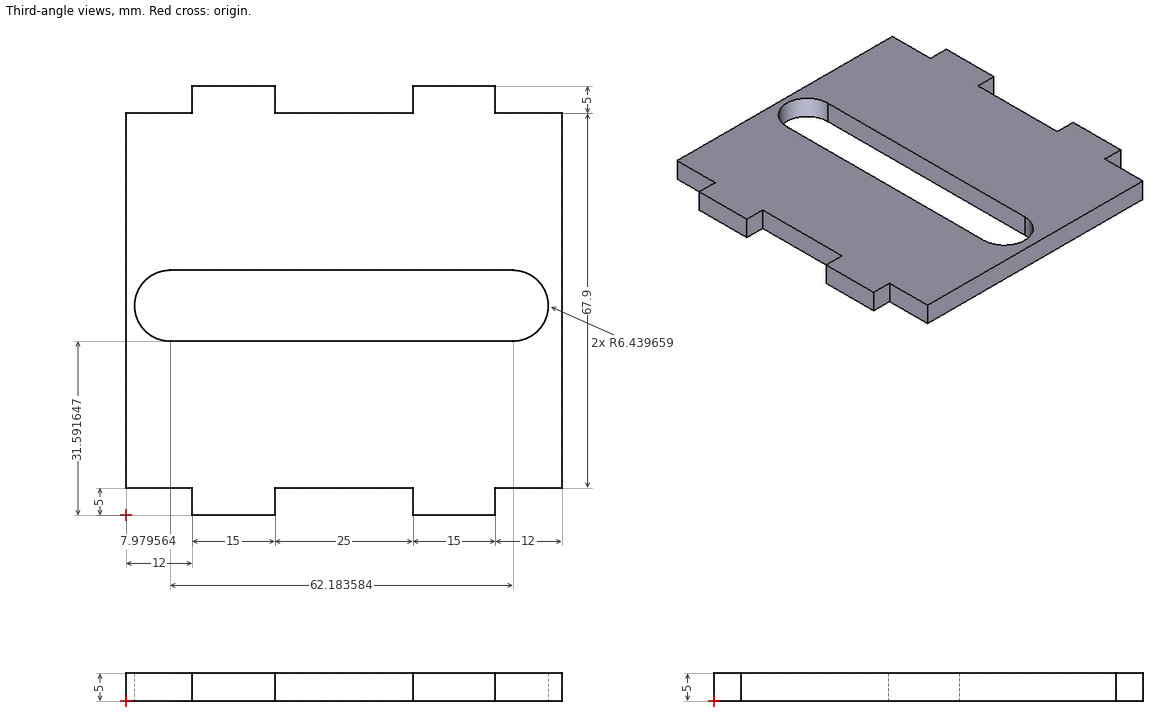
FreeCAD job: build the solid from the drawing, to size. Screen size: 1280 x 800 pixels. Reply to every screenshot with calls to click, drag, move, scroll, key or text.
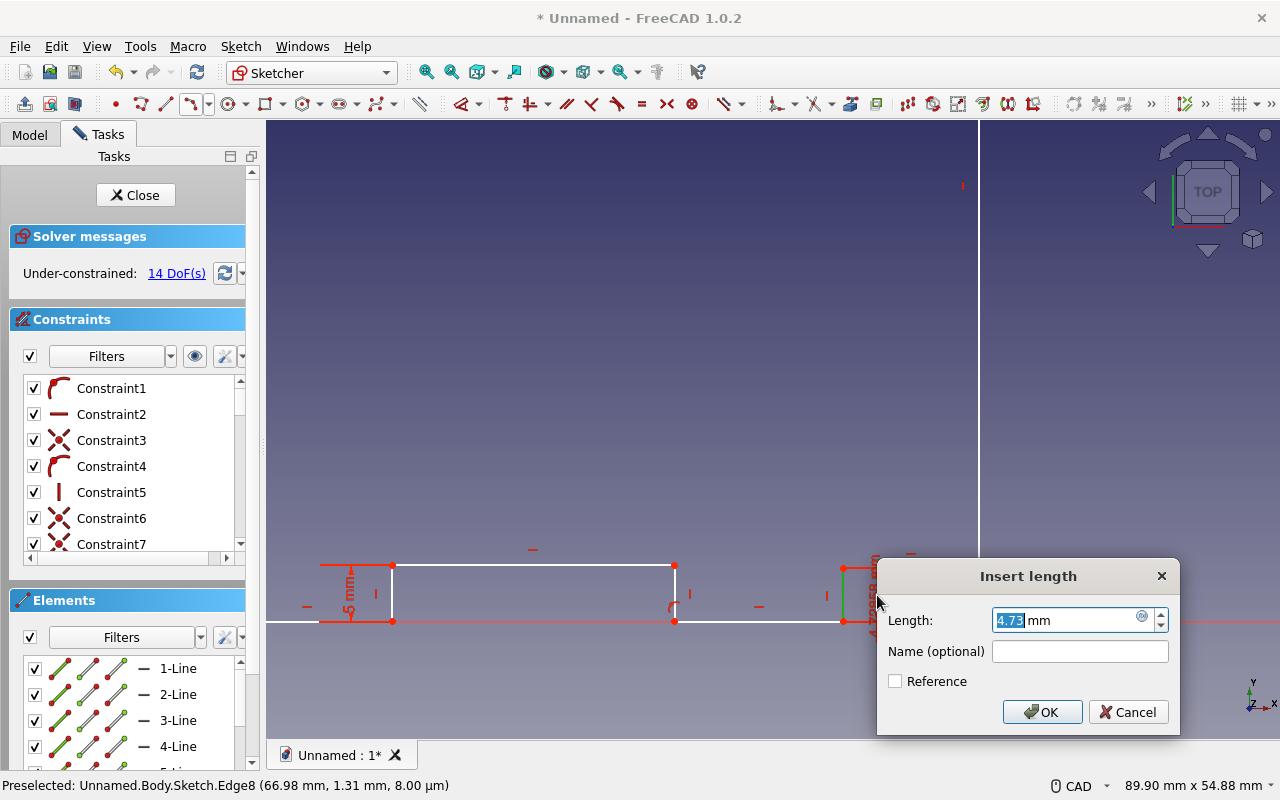
text(5)
key(Return)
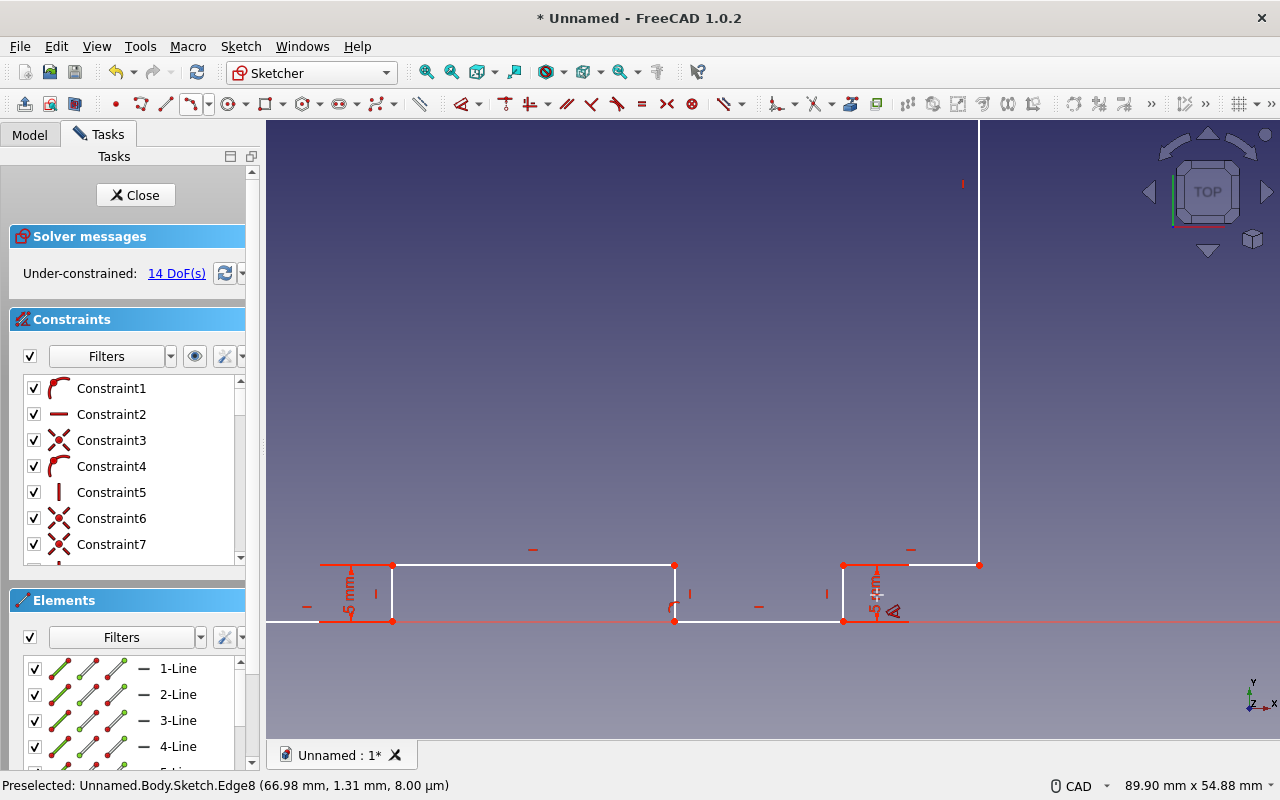
scroll(844, 631, down, 4)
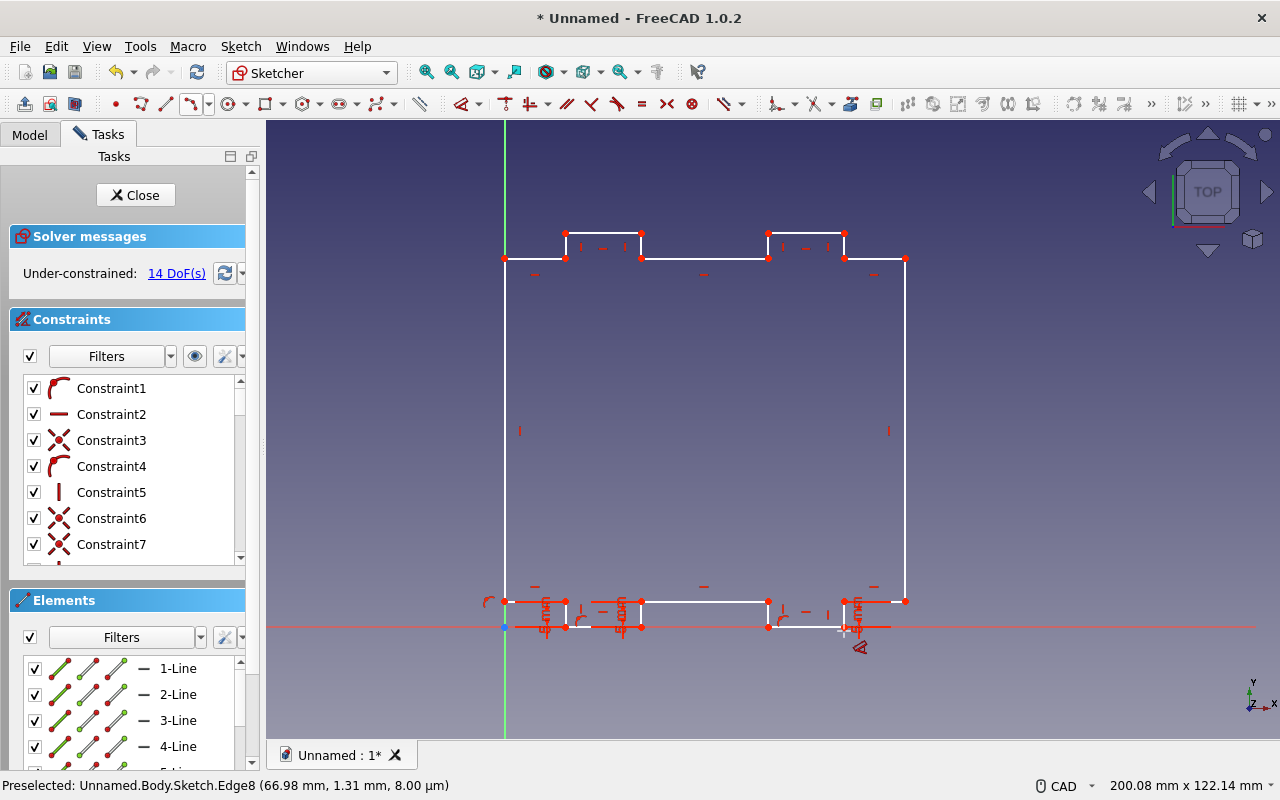
scroll(844, 251, up, 3)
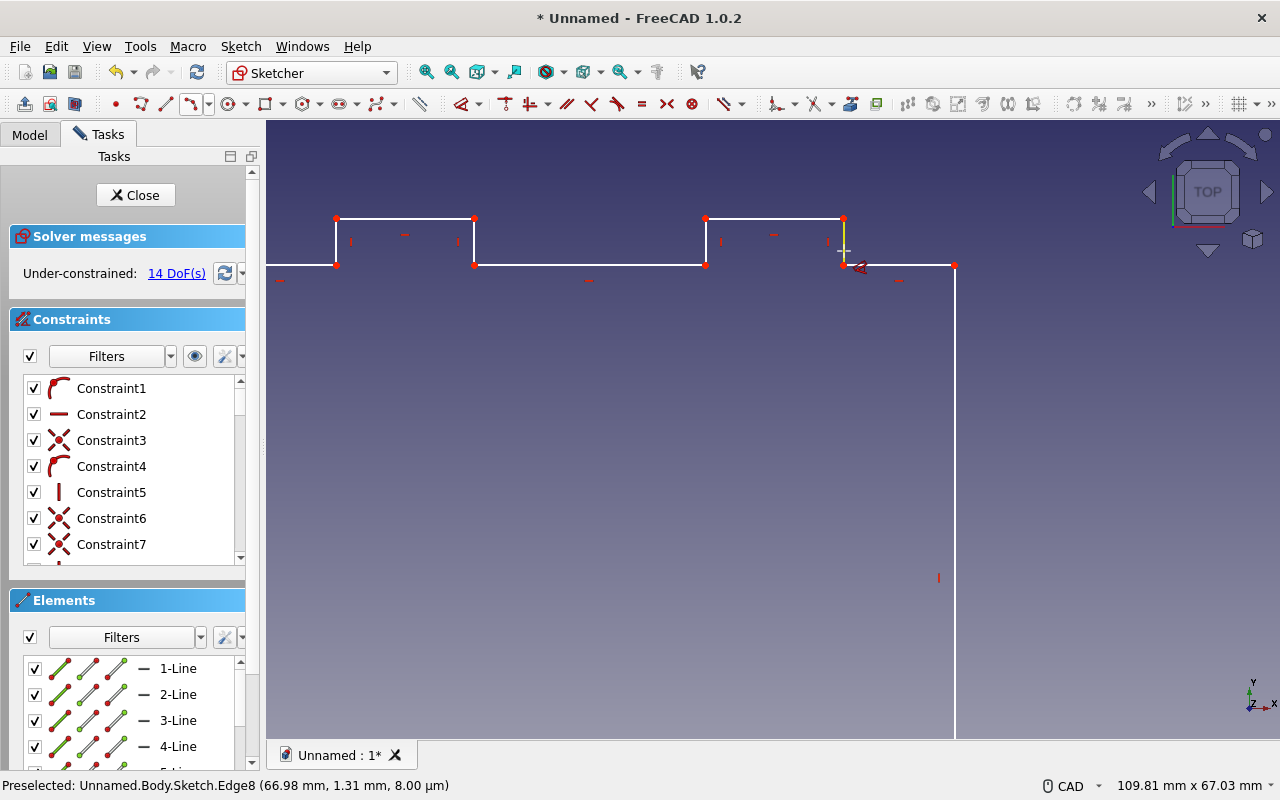
click(844, 251)
click(878, 242)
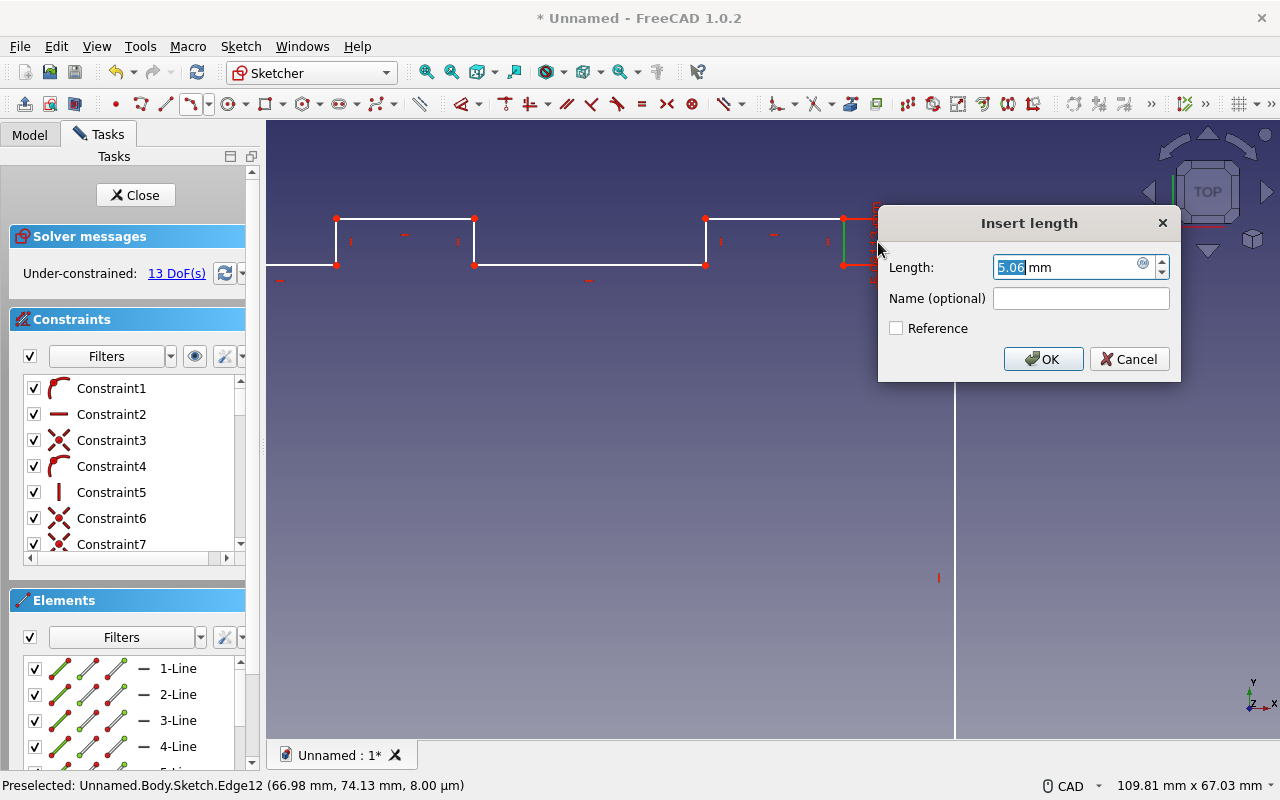
text(5)
key(Return)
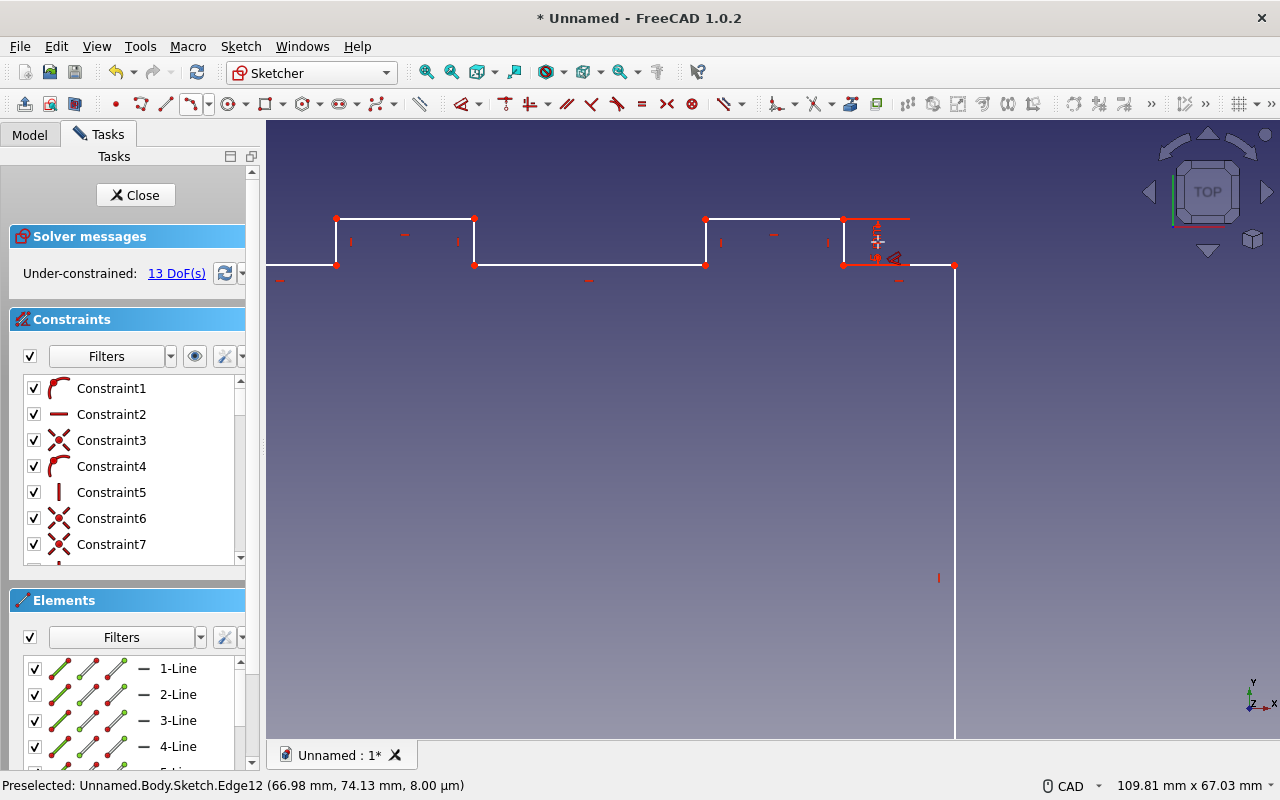
click(706, 233)
click(740, 242)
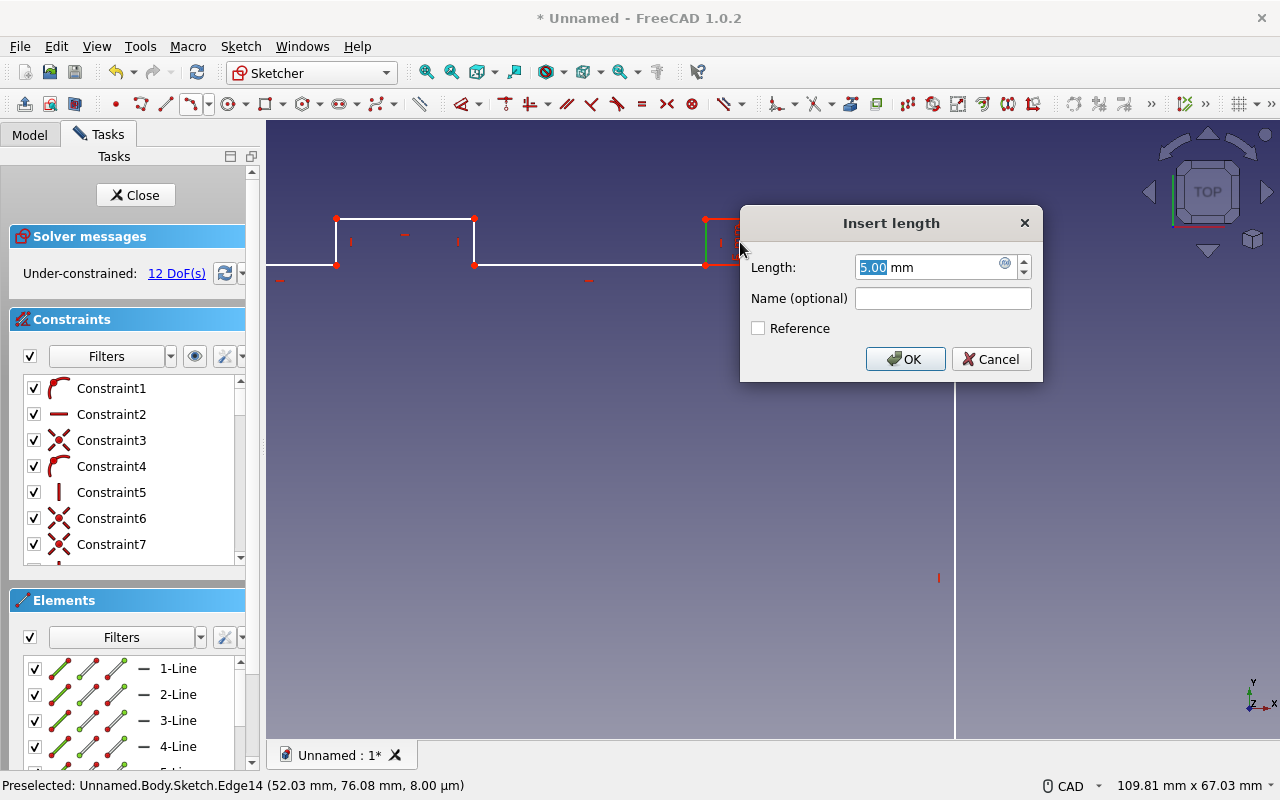
text(5)
key(Return)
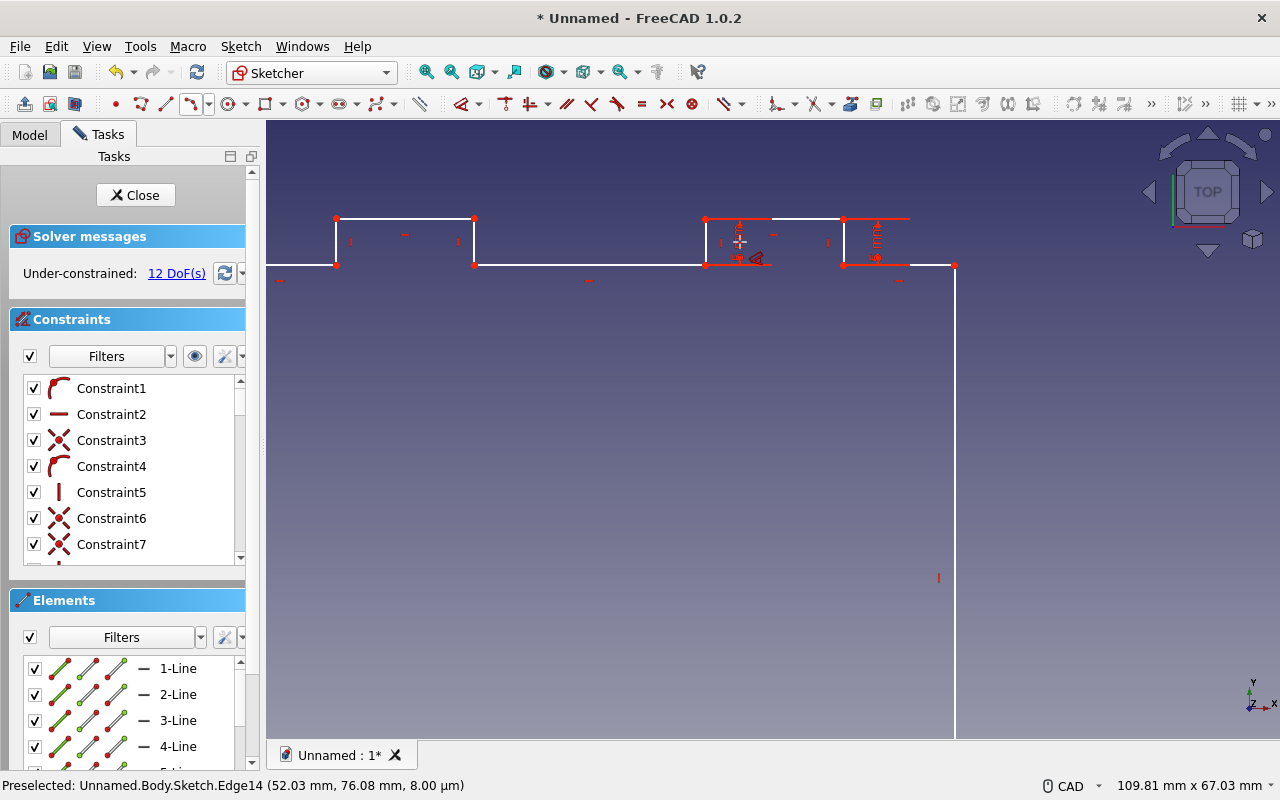
click(474, 251)
click(440, 242)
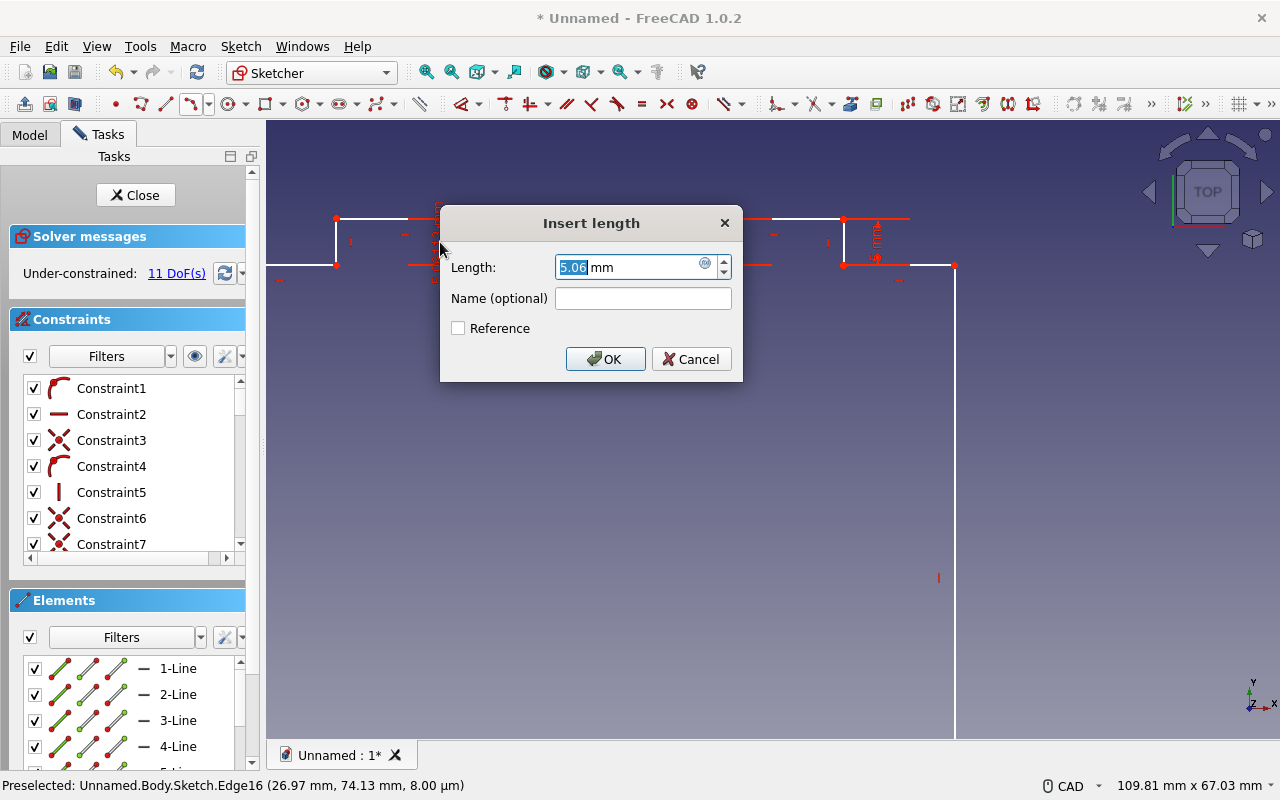
text(5)
key(Return)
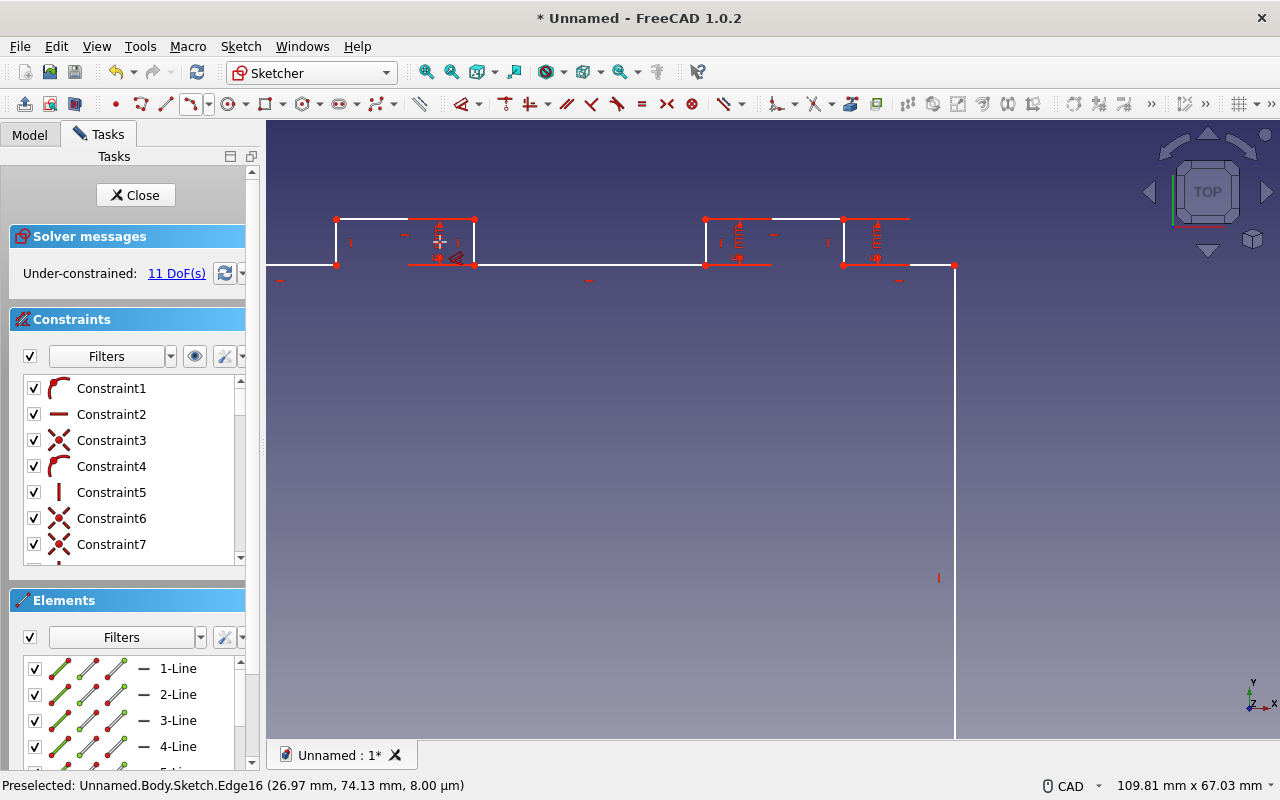
click(336, 233)
click(302, 242)